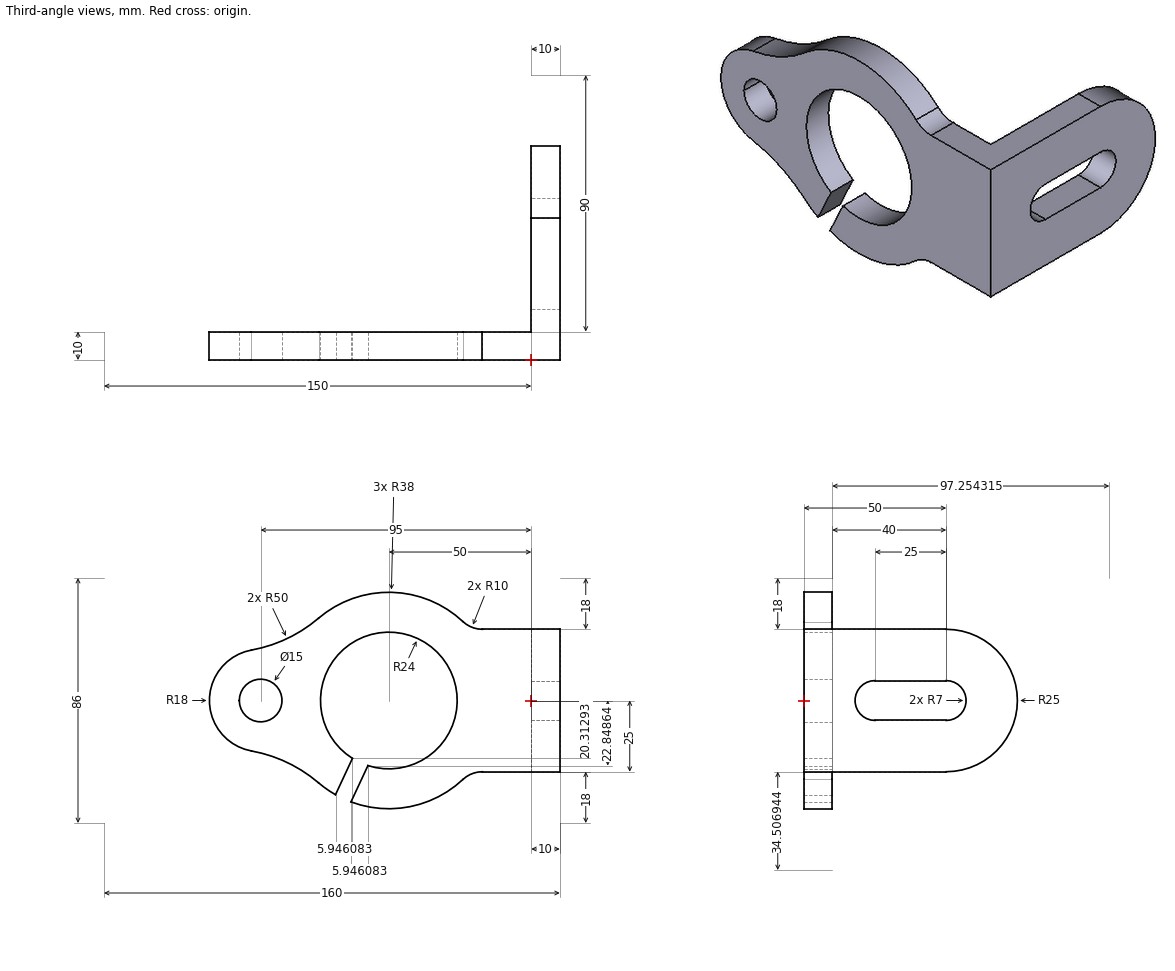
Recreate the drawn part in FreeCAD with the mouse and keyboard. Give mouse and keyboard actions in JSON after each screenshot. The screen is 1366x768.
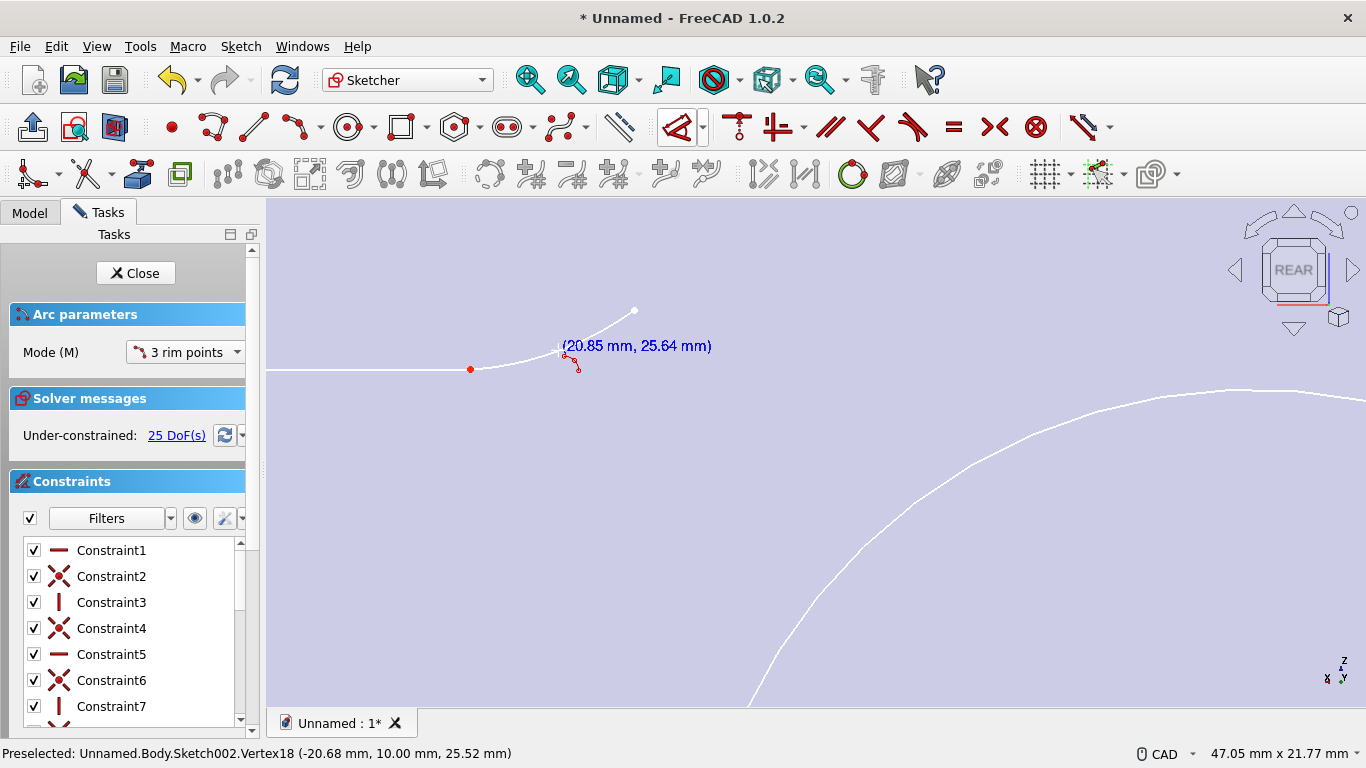
{"action": "scroll", "coordinate": [557, 354], "scroll_direction": "down", "scroll_amount": 9}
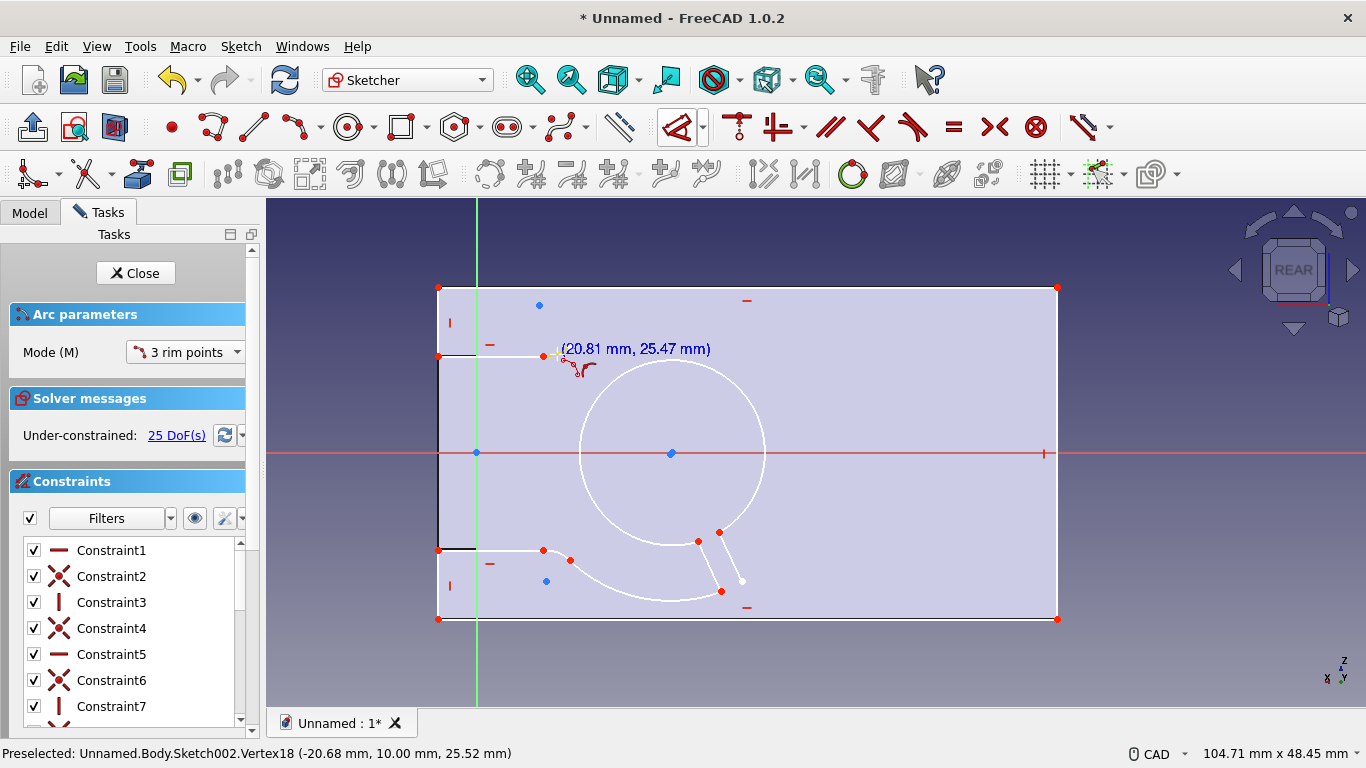
{"action": "left_click", "coordinate": [570, 347]}
{"action": "left_click", "coordinate": [765, 341]}
{"action": "left_click", "coordinate": [667, 306]}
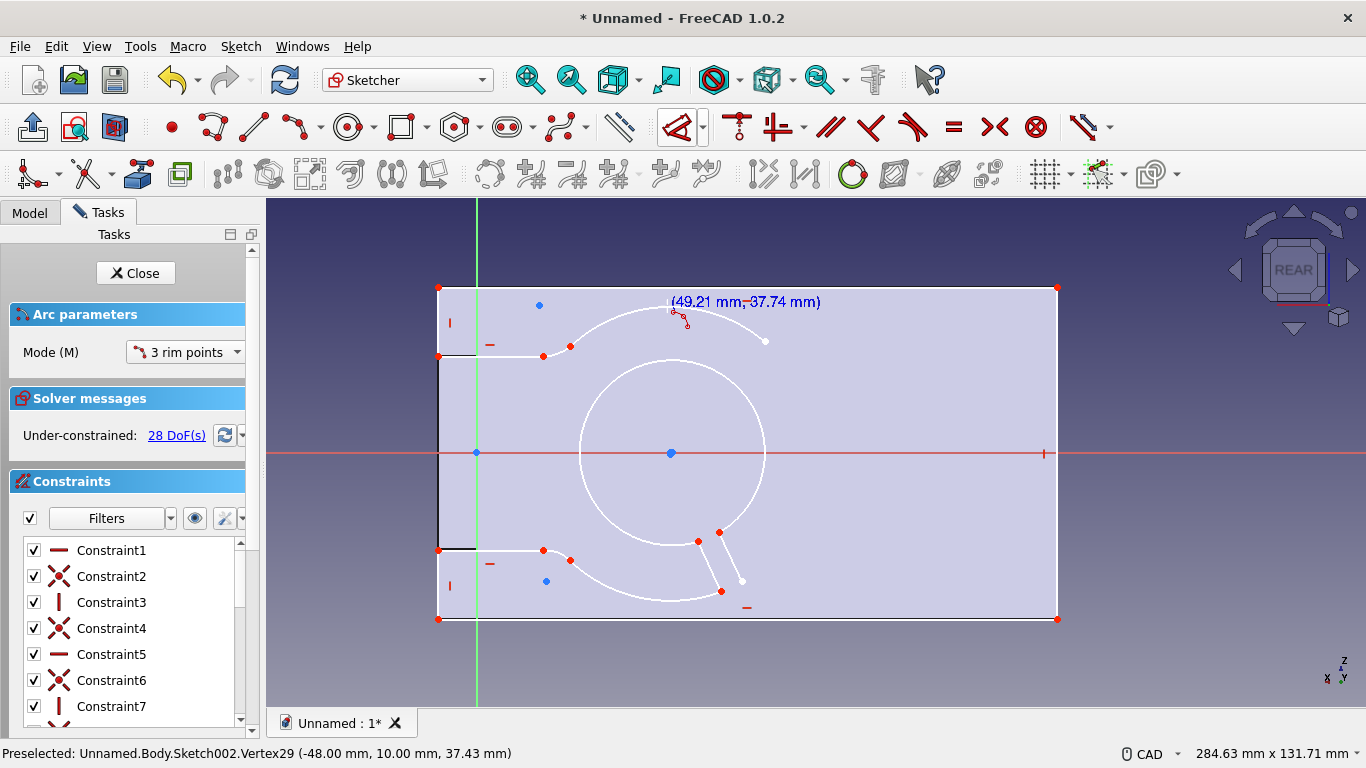
{"action": "left_click", "coordinate": [765, 342]}
{"action": "left_click", "coordinate": [856, 384]}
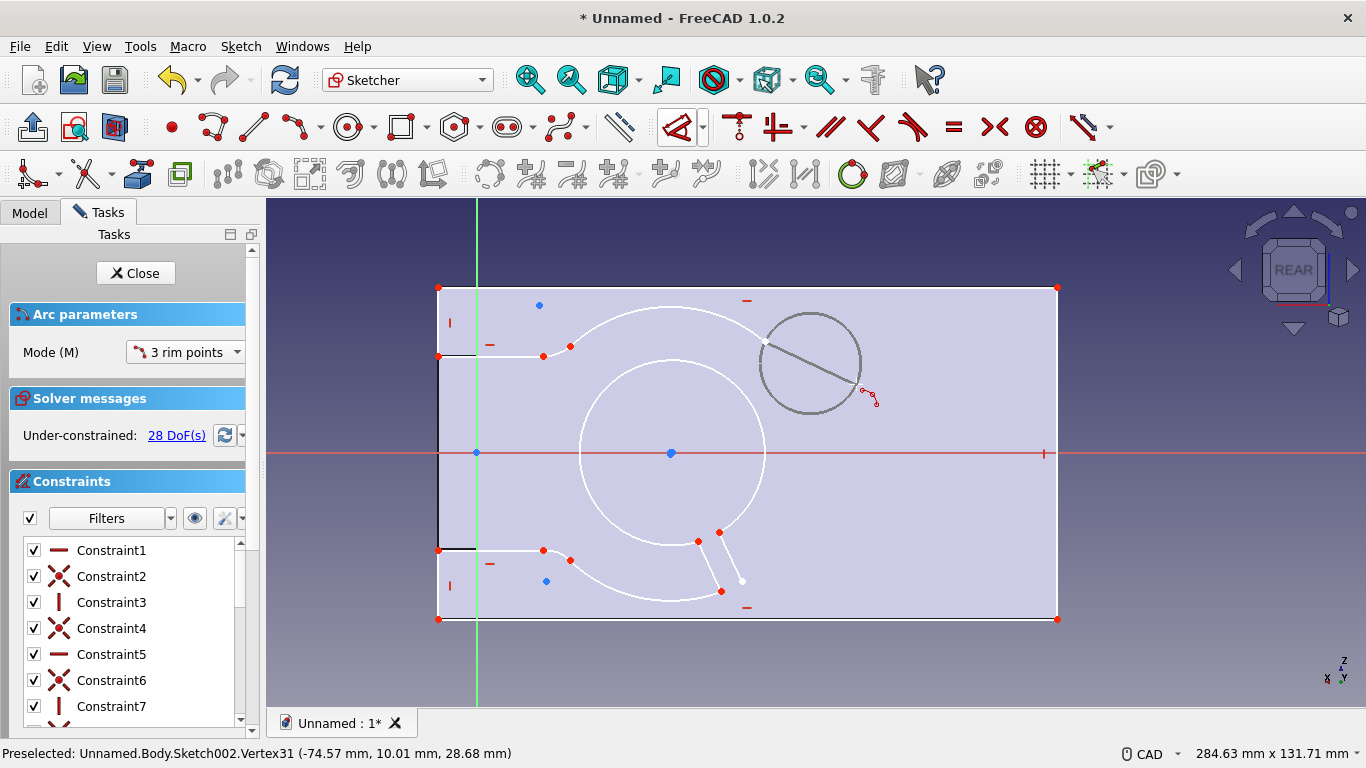
{"action": "scroll", "coordinate": [808, 369], "scroll_direction": "up", "scroll_amount": 5}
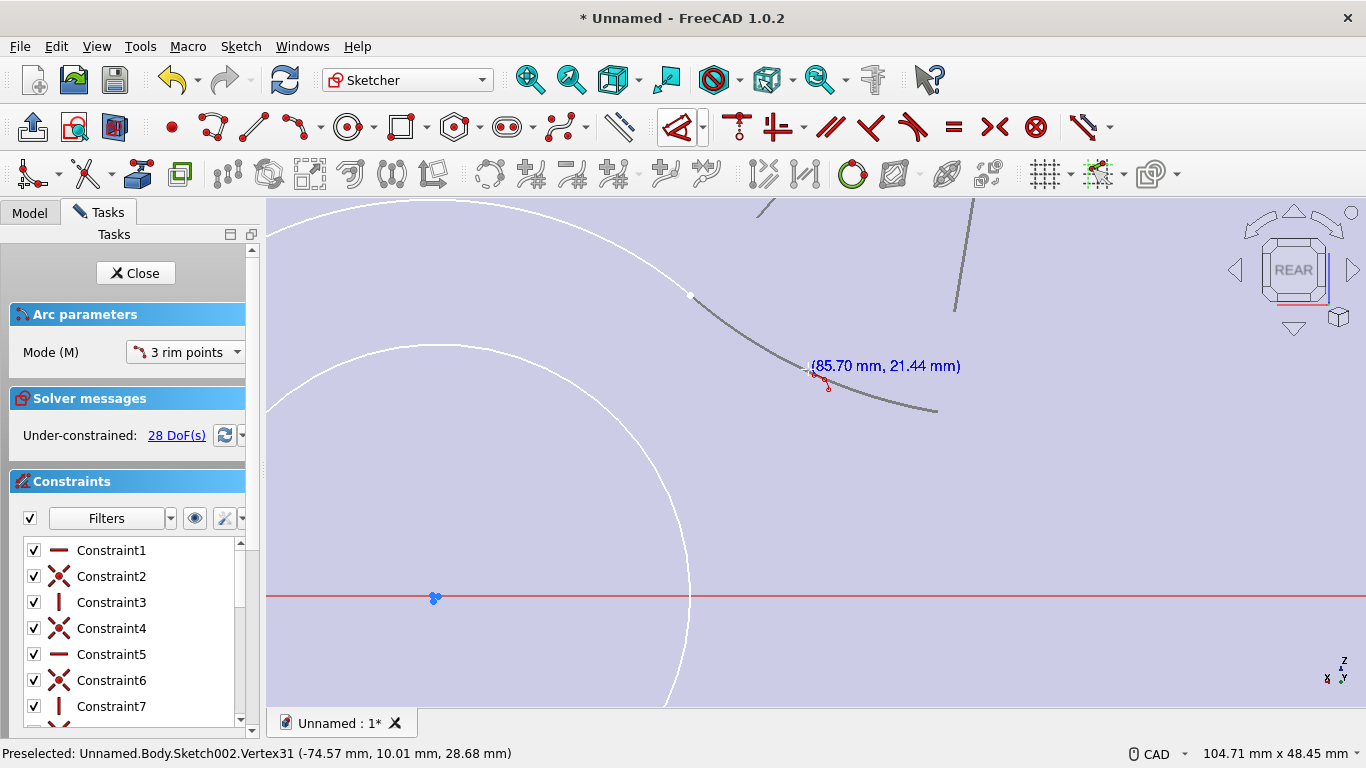
{"action": "left_click", "coordinate": [807, 368]}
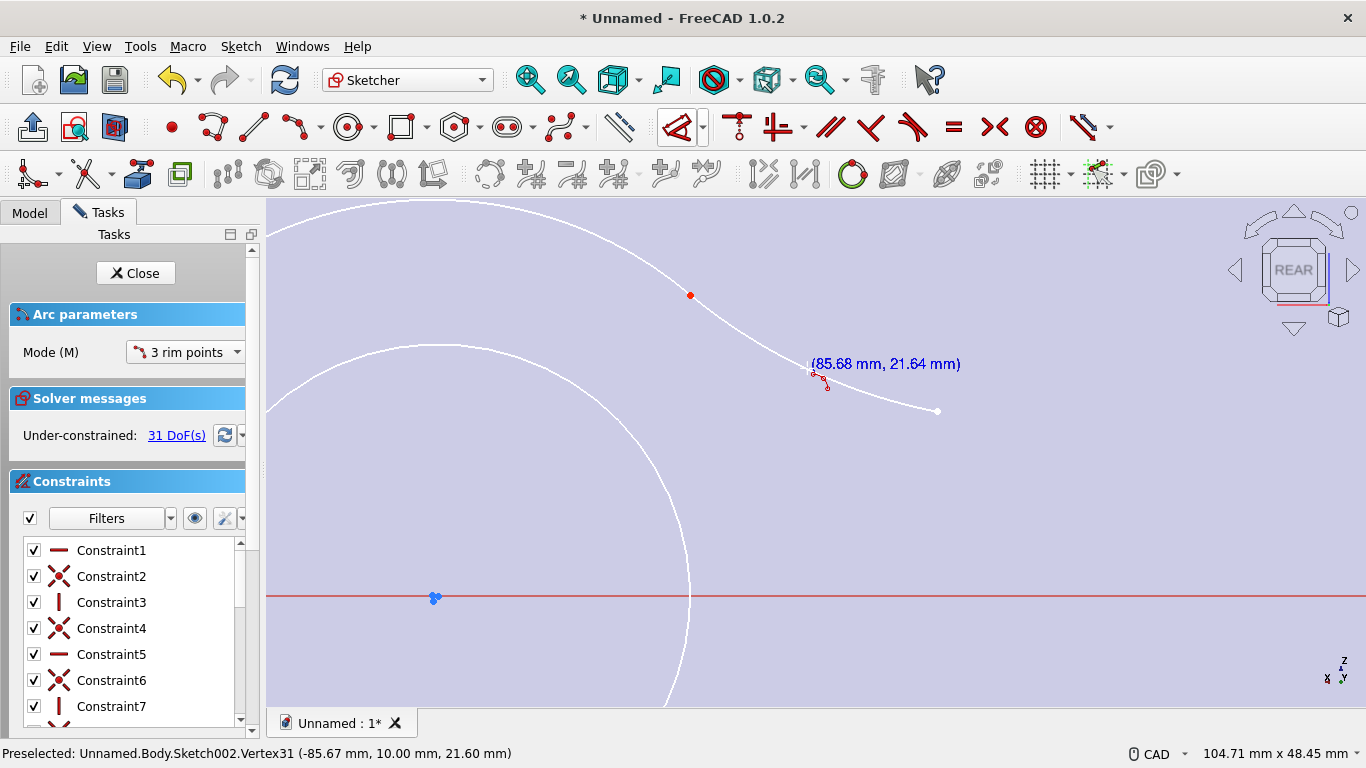
{"action": "left_click", "coordinate": [938, 412]}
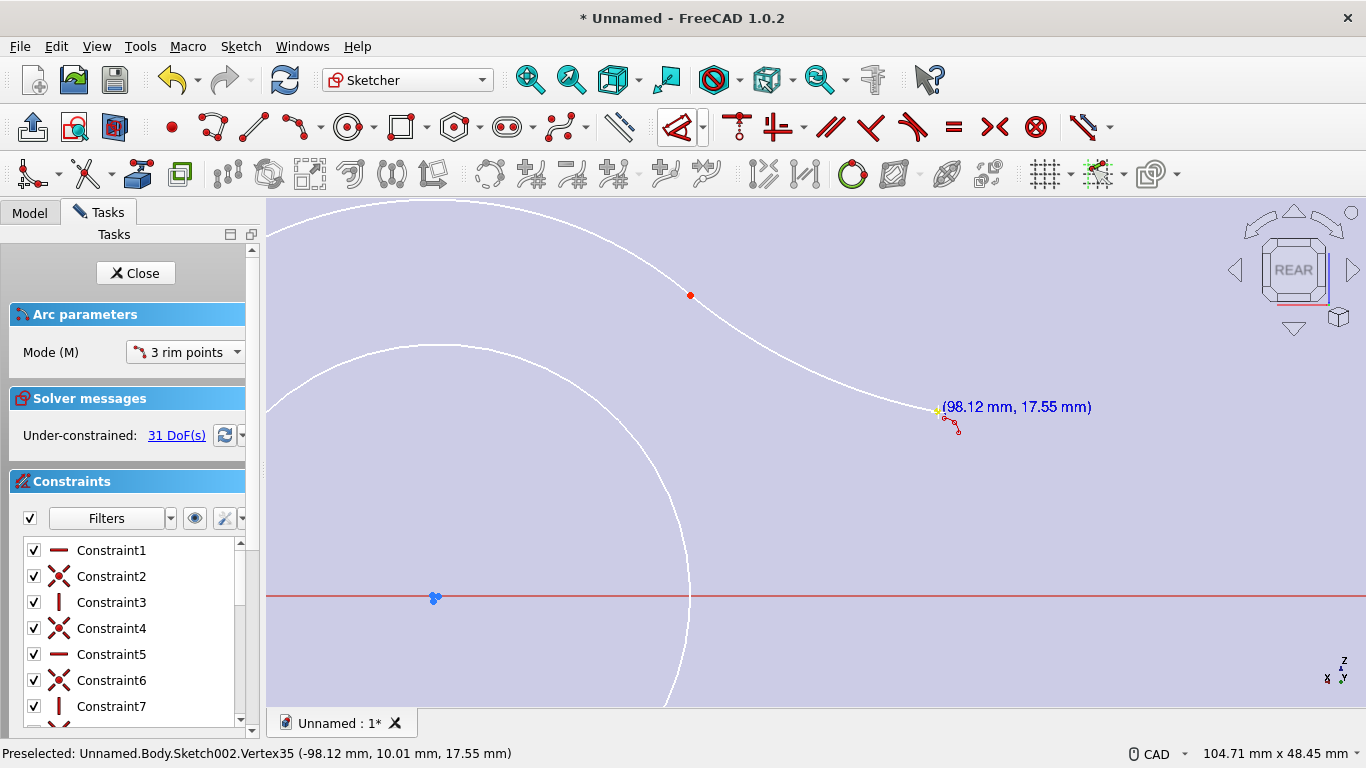
{"action": "scroll", "coordinate": [809, 369], "scroll_direction": "down", "scroll_amount": 5}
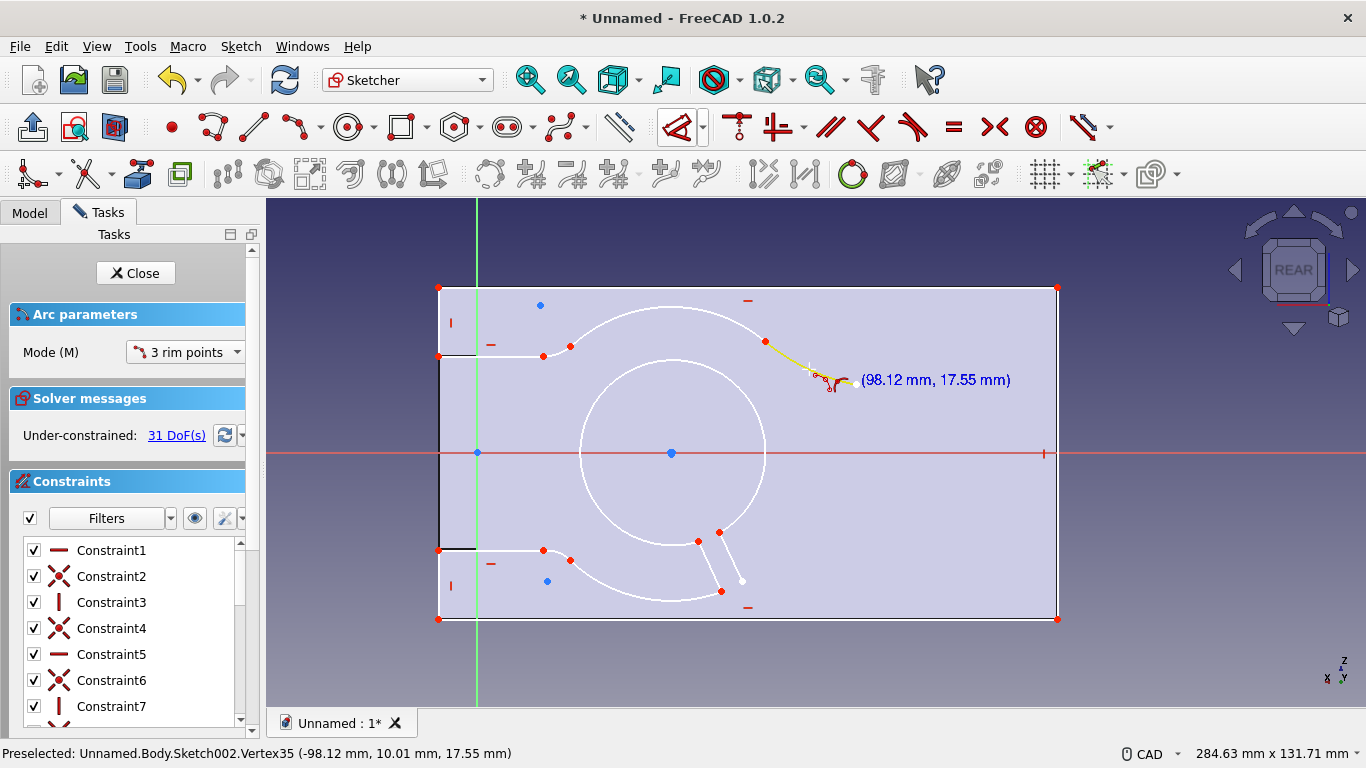
{"action": "left_click", "coordinate": [857, 521]}
{"action": "left_click", "coordinate": [911, 472]}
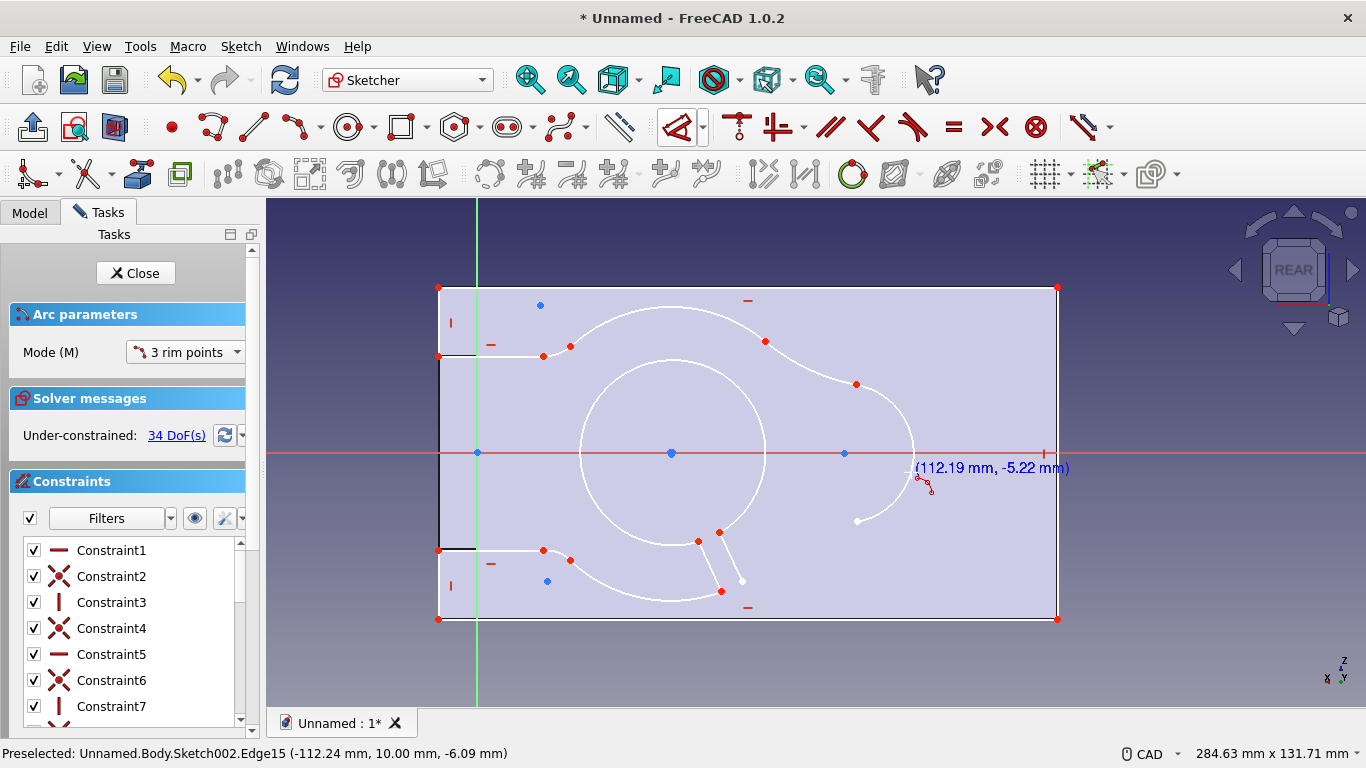
{"action": "left_click", "coordinate": [857, 522]}
{"action": "left_click", "coordinate": [766, 564]}